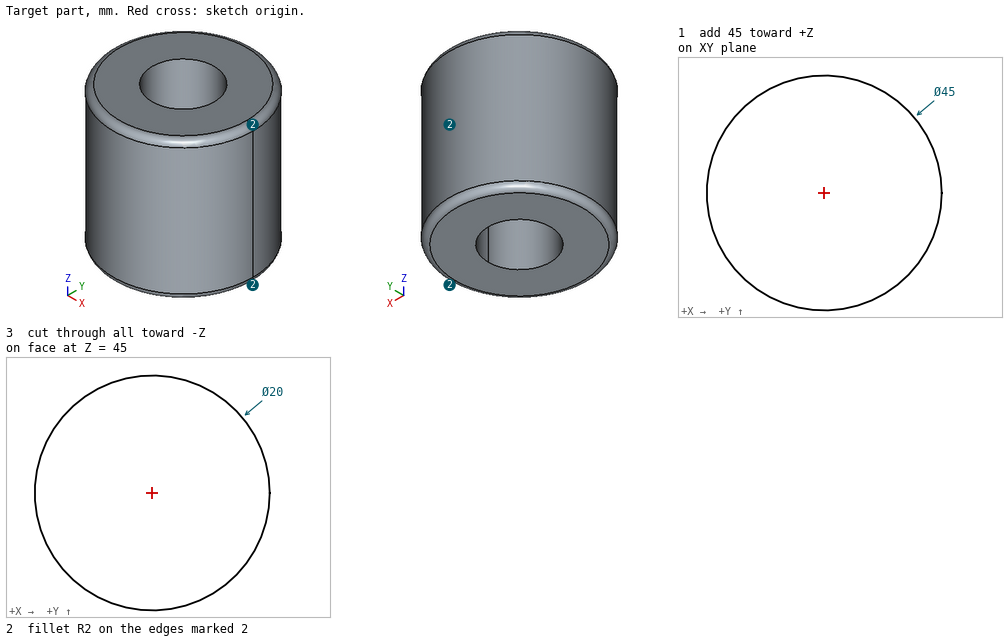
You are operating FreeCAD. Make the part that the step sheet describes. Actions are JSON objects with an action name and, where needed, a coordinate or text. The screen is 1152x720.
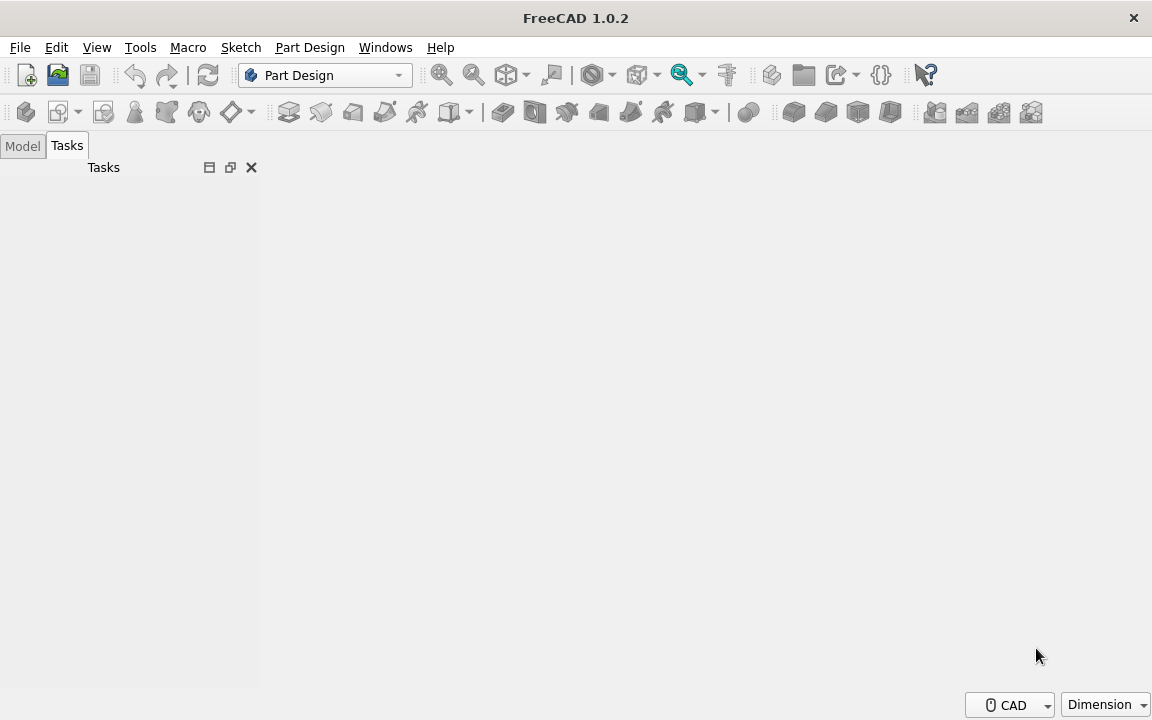
{"action": "left_click", "coordinate": [26, 76]}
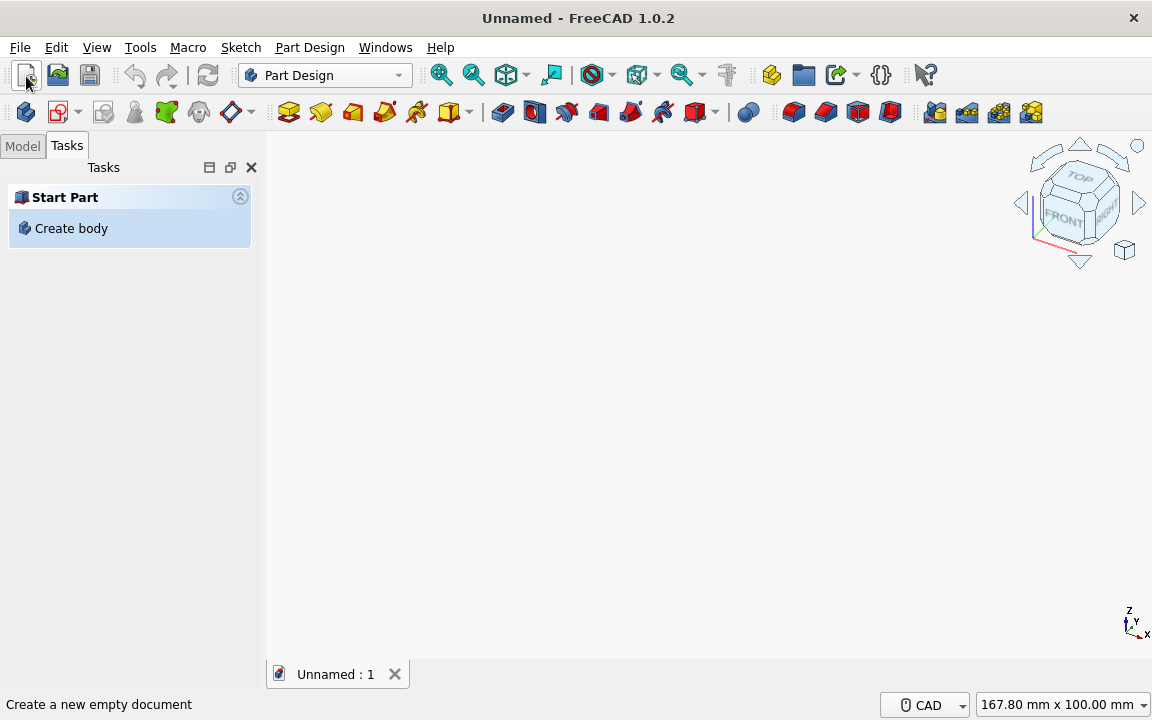
{"action": "left_click", "coordinate": [58, 112]}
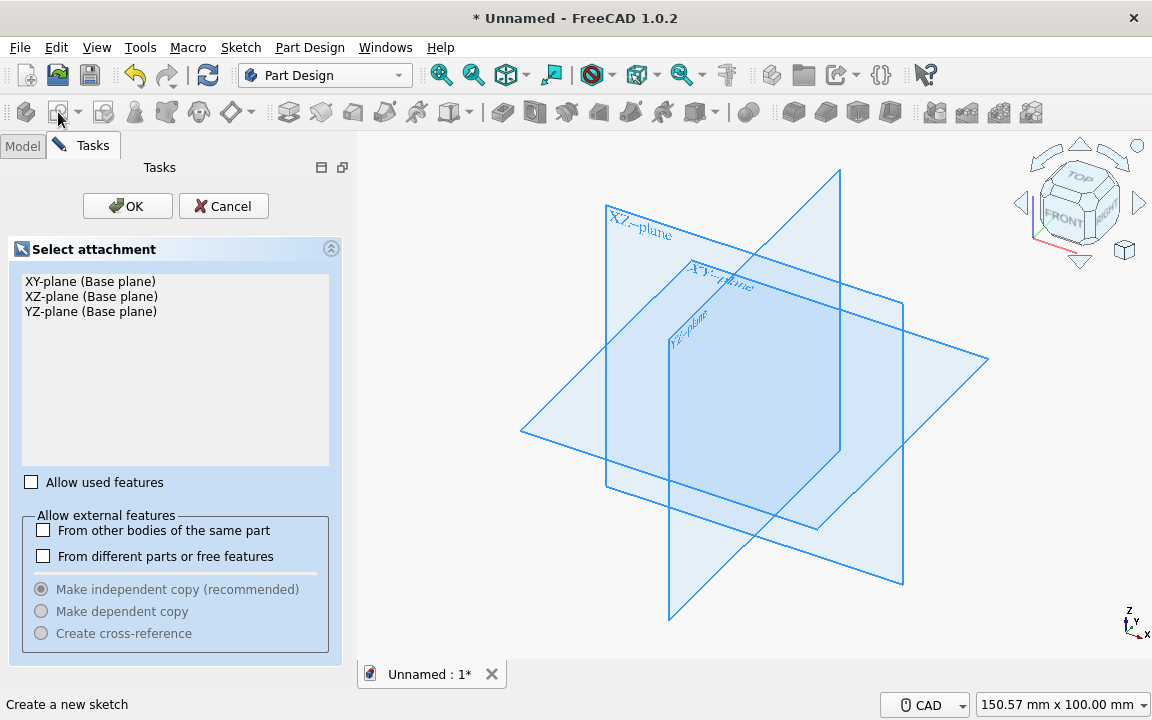
{"action": "left_click", "coordinate": [82, 282]}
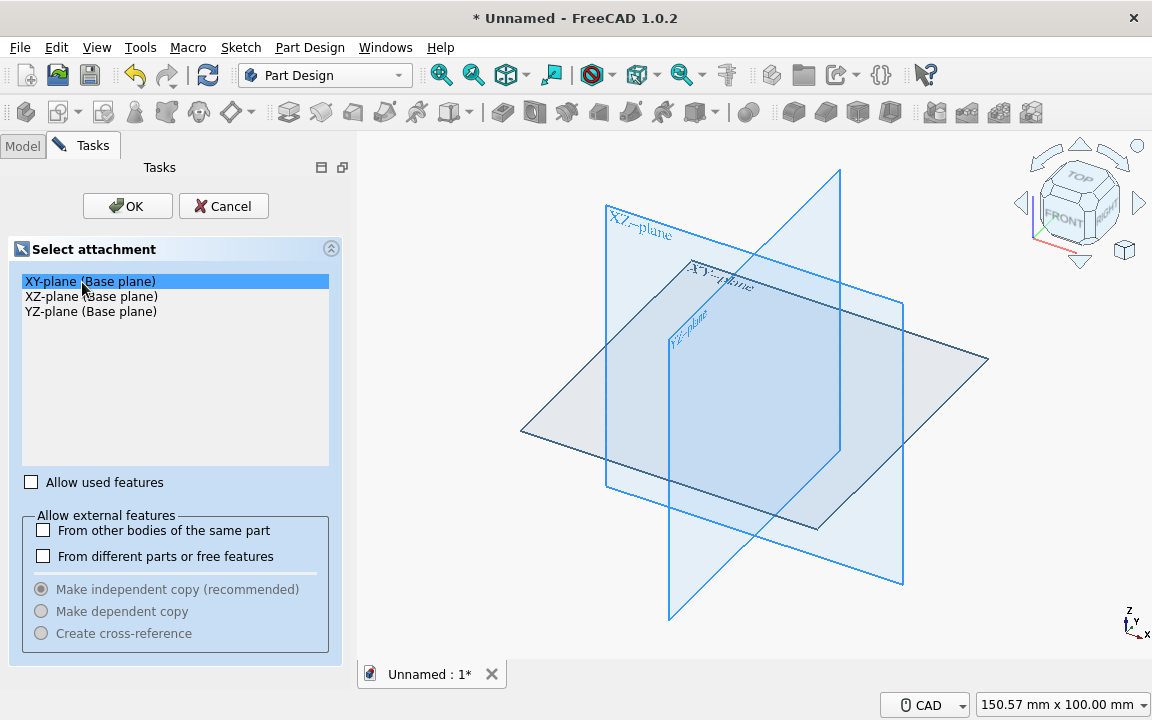
{"action": "left_click", "coordinate": [128, 206]}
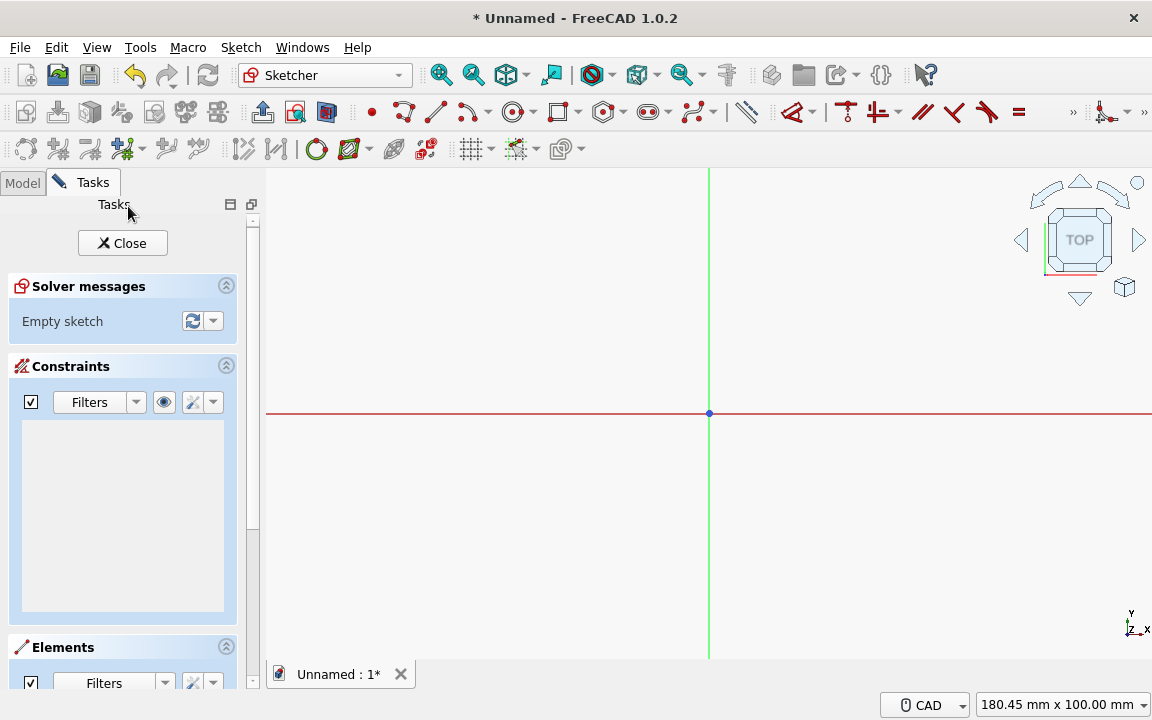
{"action": "scroll", "coordinate": [848, 413], "scroll_direction": "up", "scroll_amount": 2}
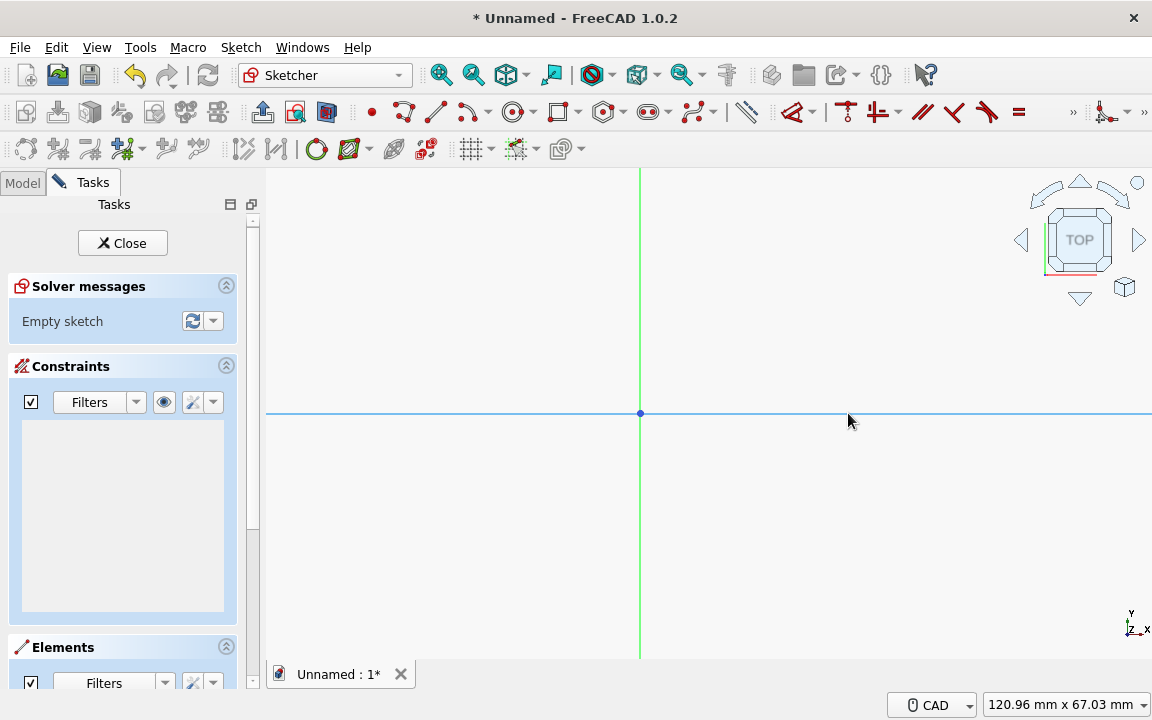
{"action": "left_click", "coordinate": [514, 112]}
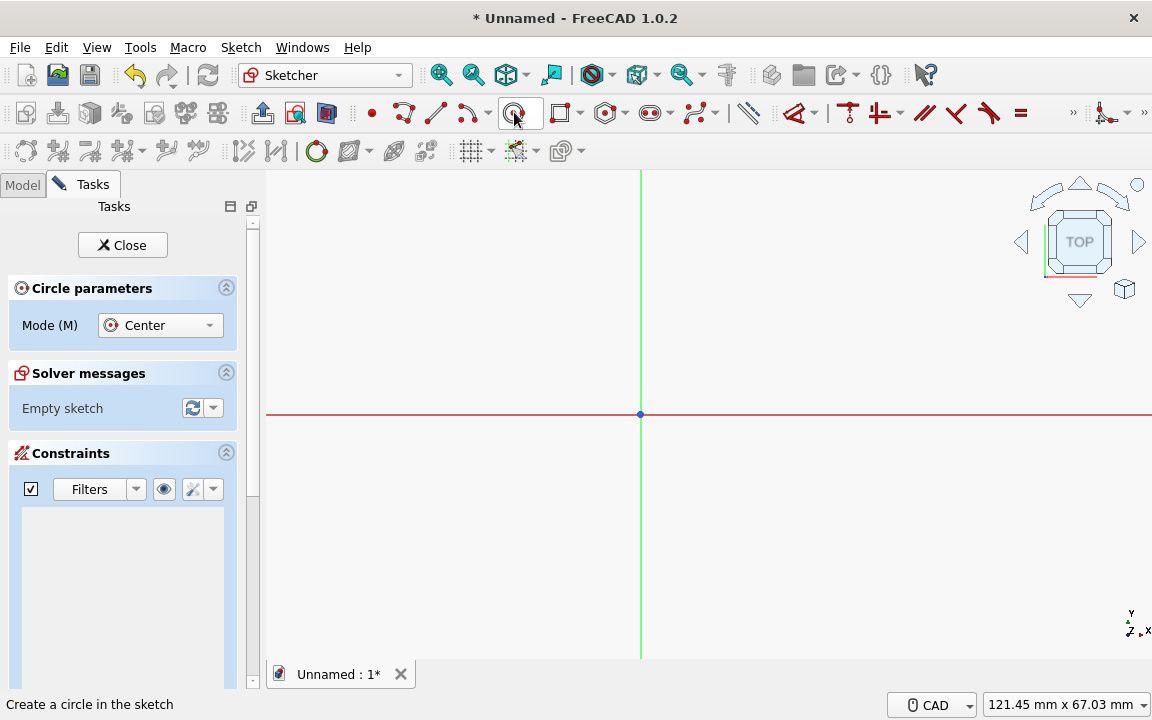
{"action": "left_click", "coordinate": [641, 414]}
{"action": "left_click", "coordinate": [757, 298]}
{"action": "key", "text": "Escape"}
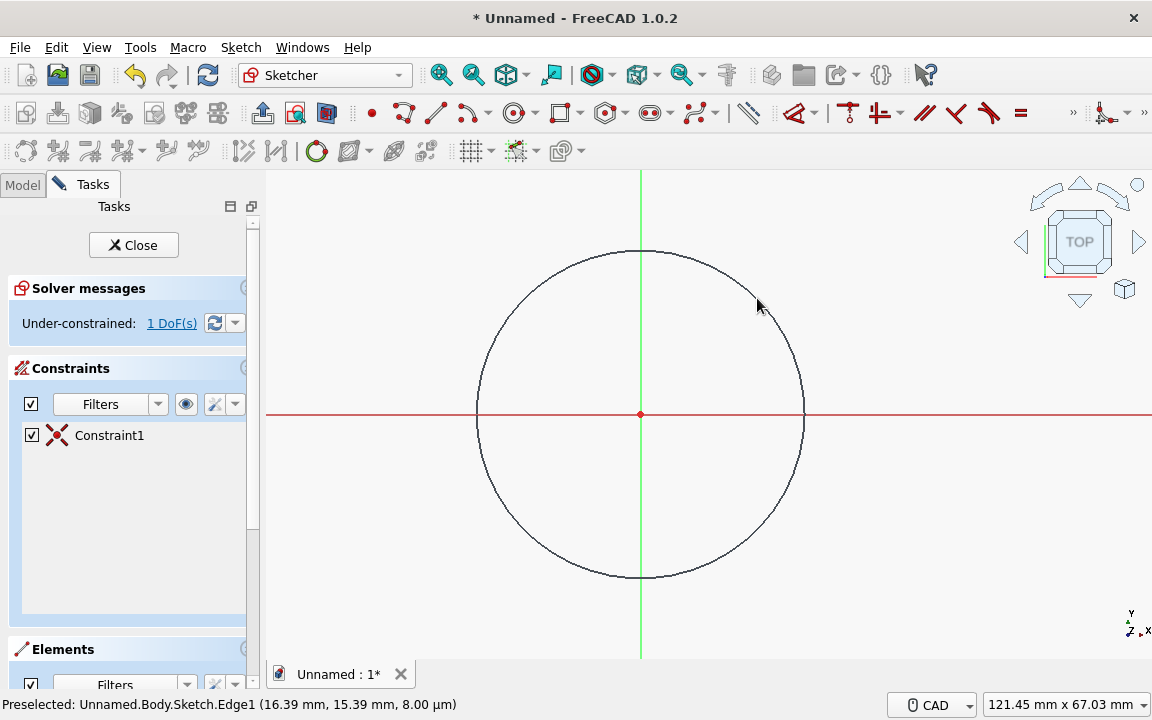
{"action": "left_click", "coordinate": [794, 114]}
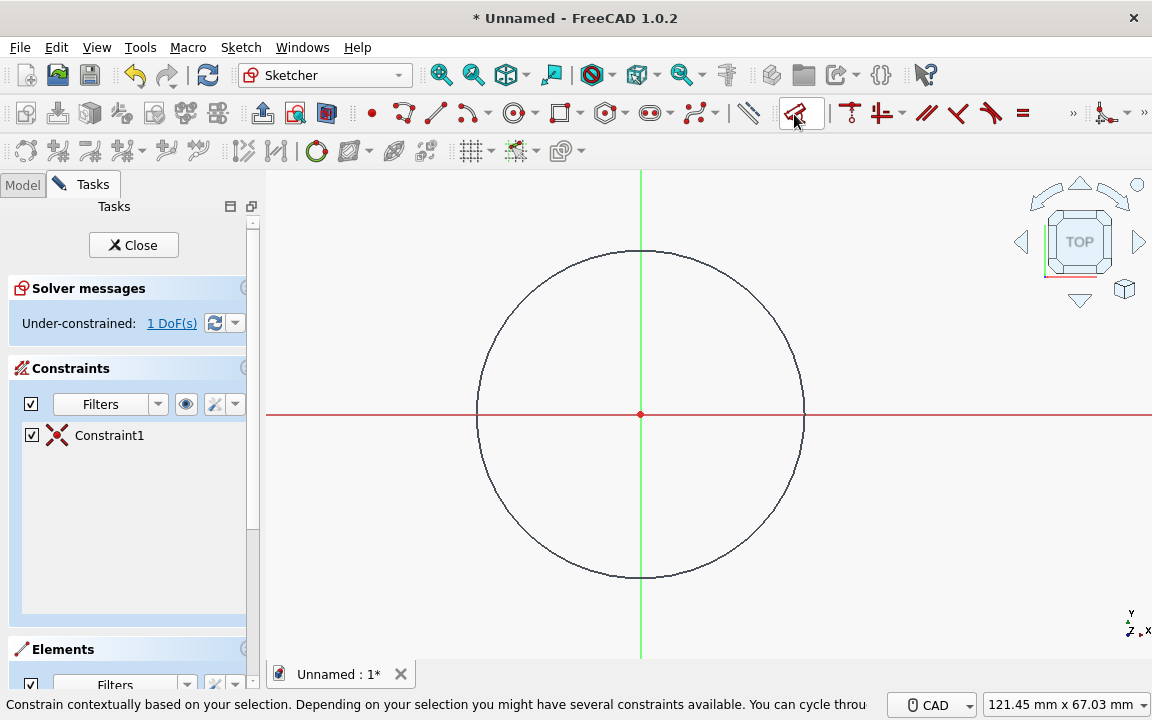
{"action": "left_click", "coordinate": [756, 298]}
{"action": "left_click", "coordinate": [779, 275]}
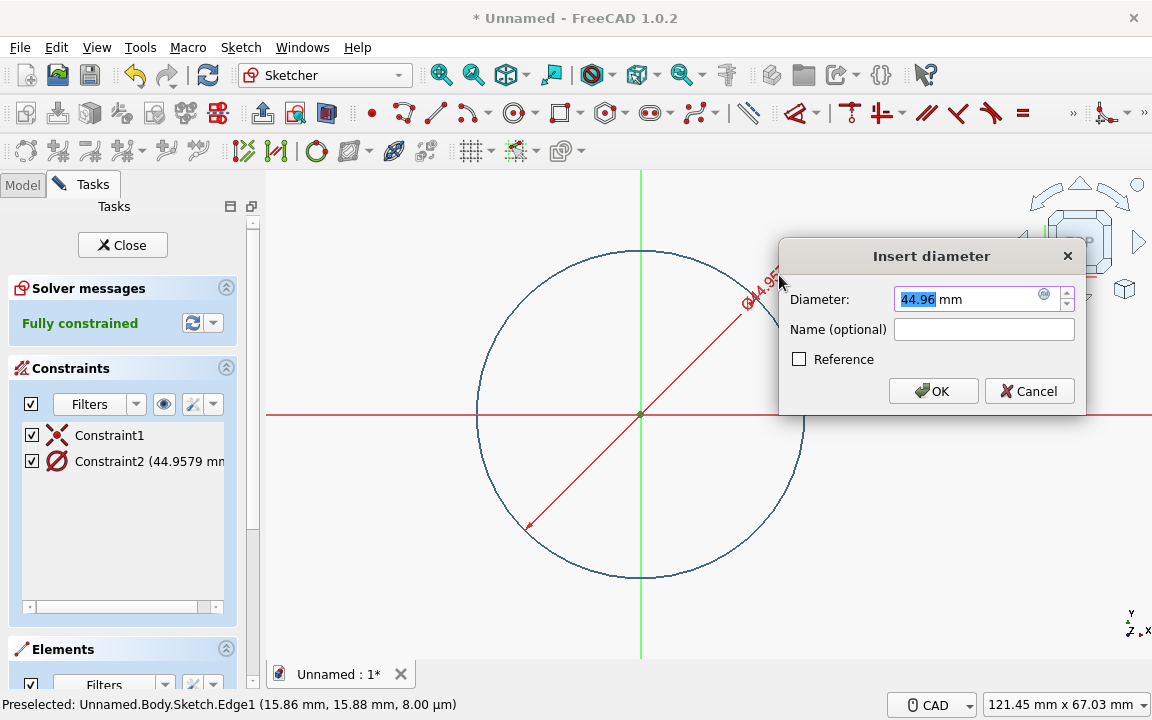
{"action": "type", "text": "45"}
{"action": "key", "text": "Return"}
{"action": "key", "text": "Escape"}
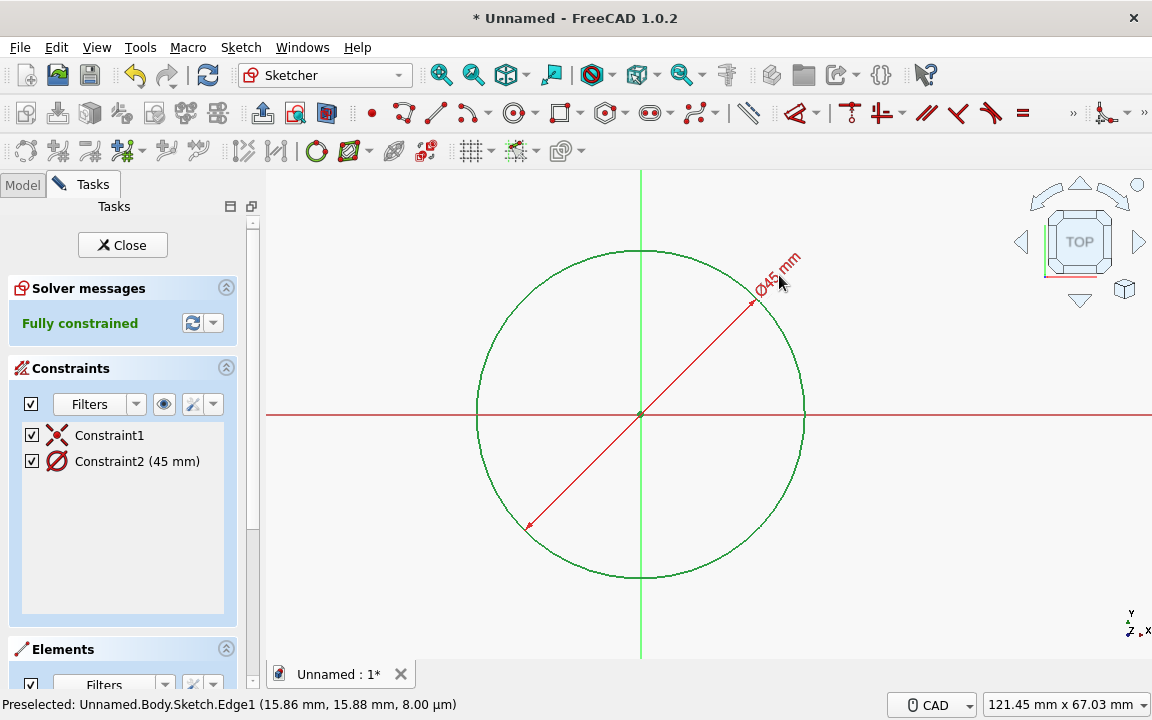
{"action": "left_click", "coordinate": [123, 245]}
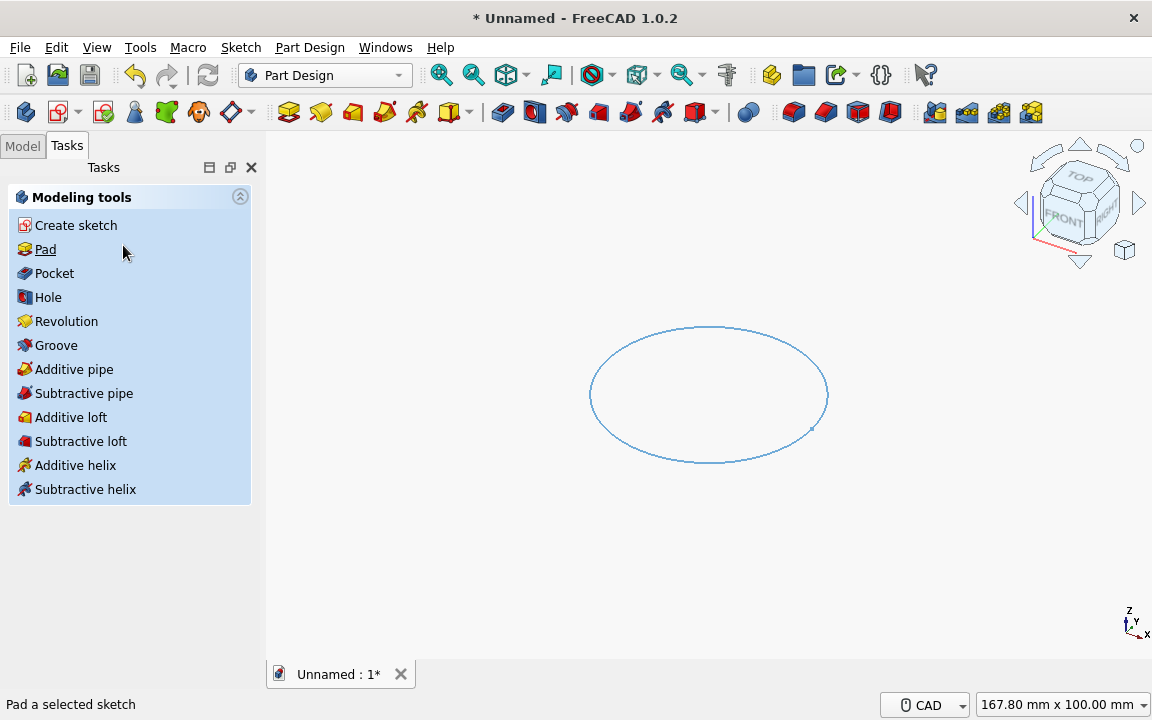
{"action": "left_click", "coordinate": [290, 112]}